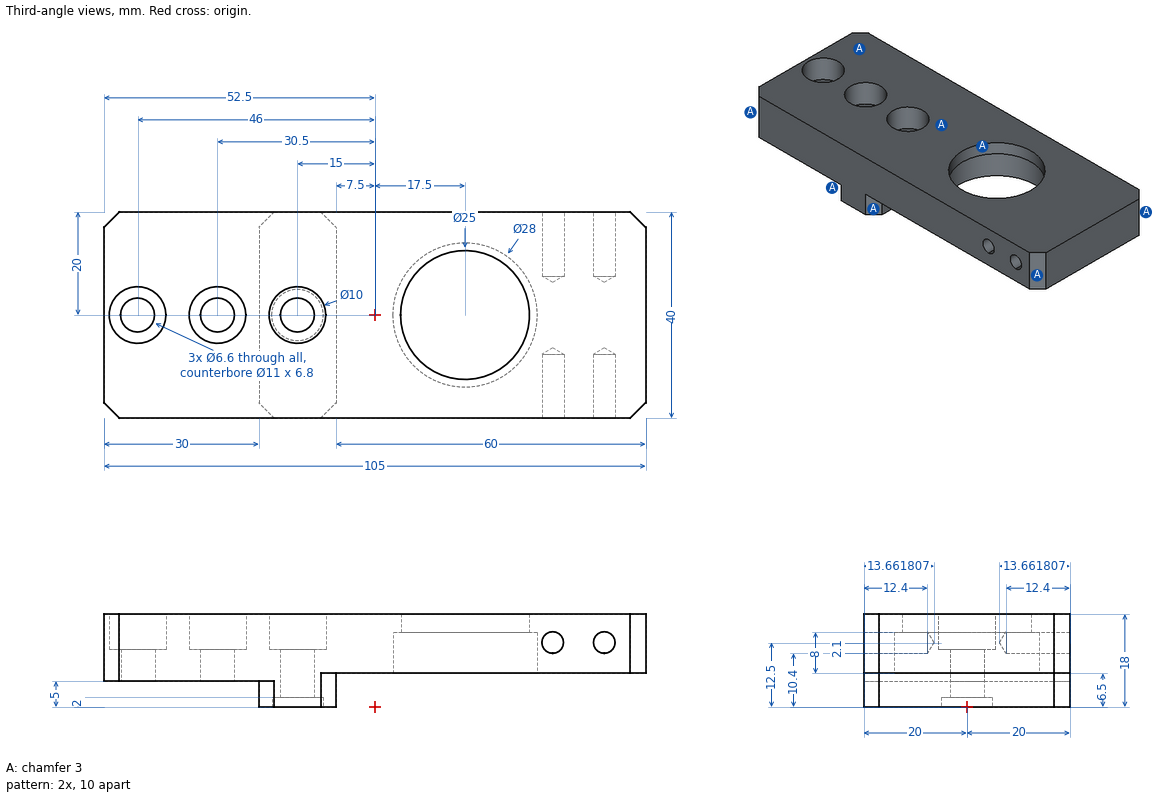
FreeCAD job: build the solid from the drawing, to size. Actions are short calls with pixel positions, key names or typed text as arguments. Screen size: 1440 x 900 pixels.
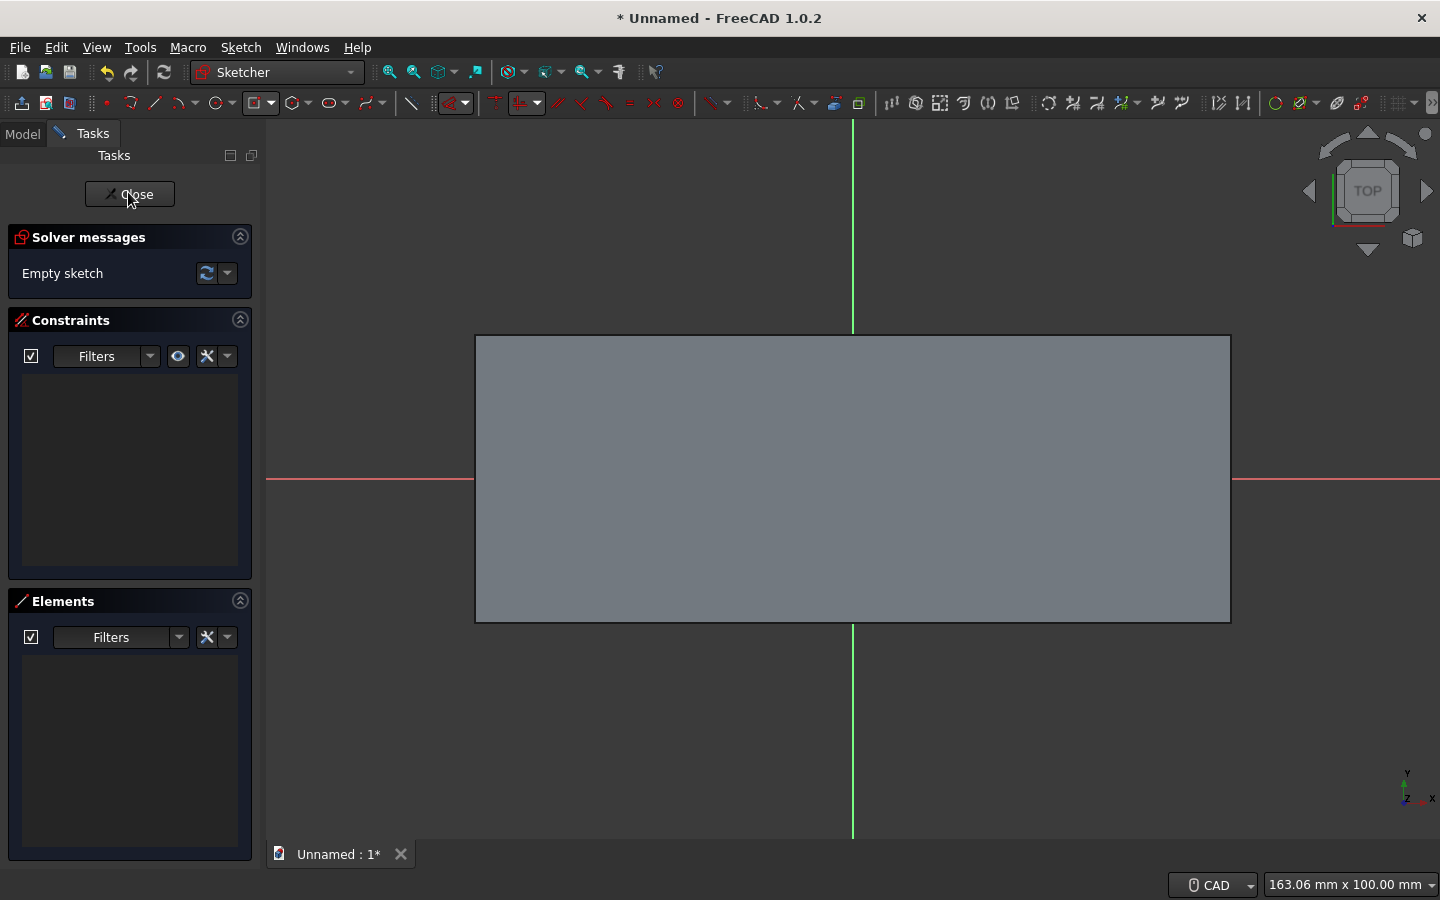
click(70, 104)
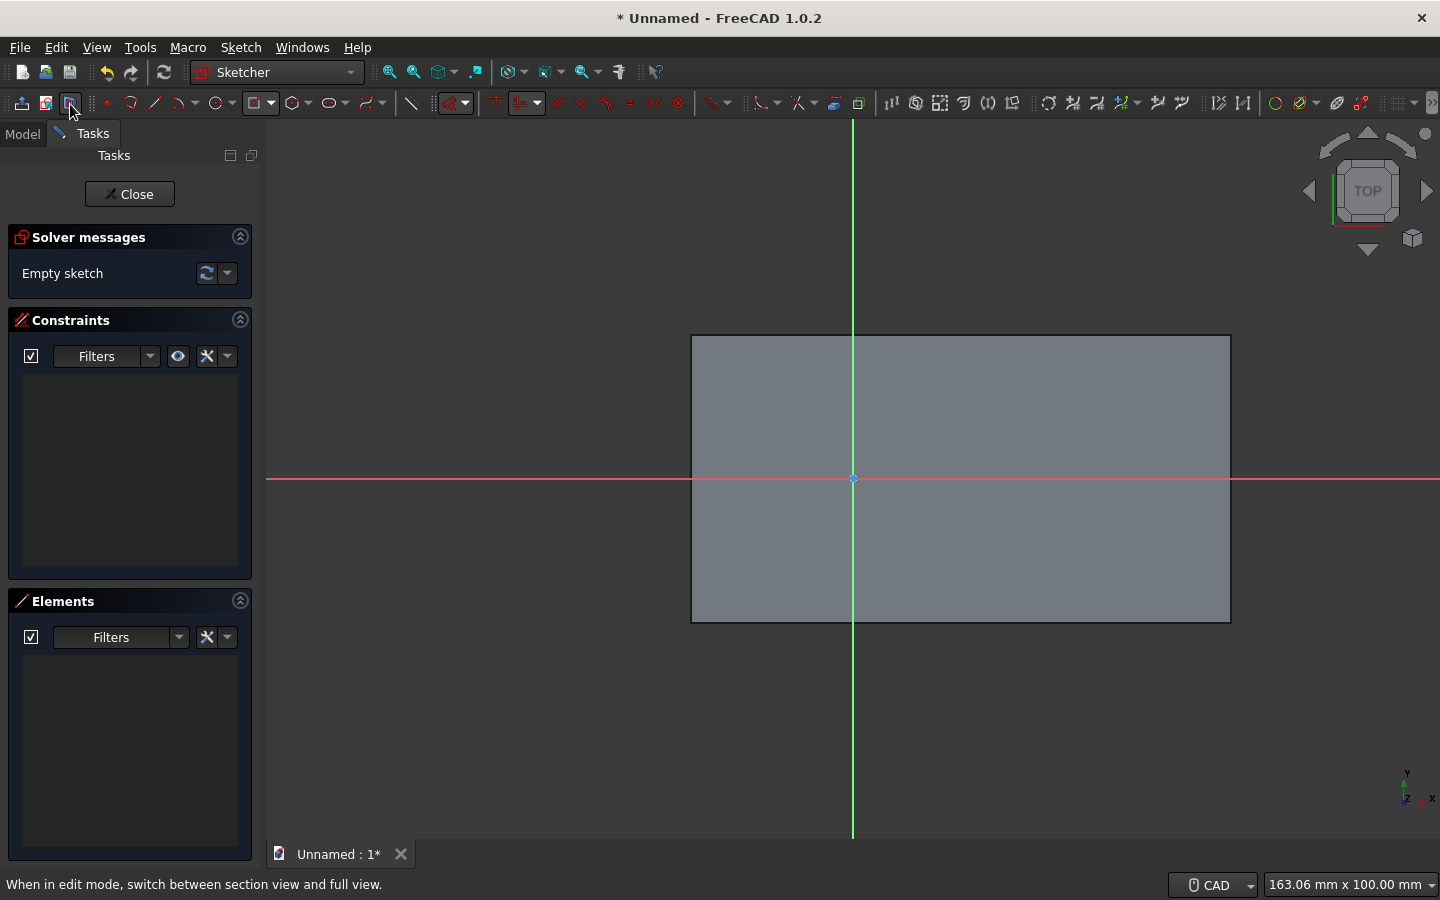
scroll(1275, 479, up, 2)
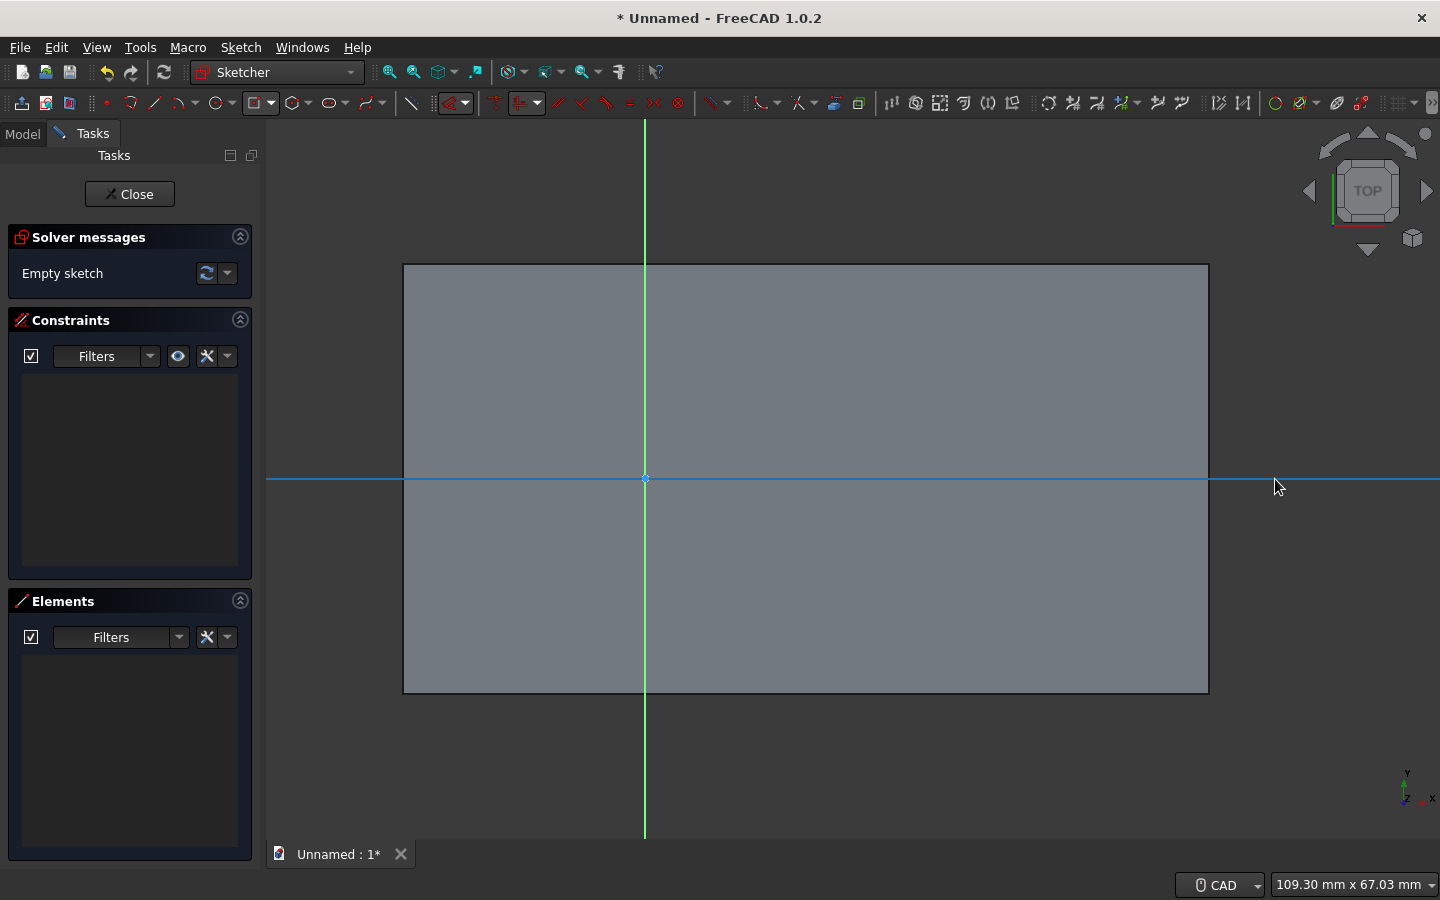
click(274, 104)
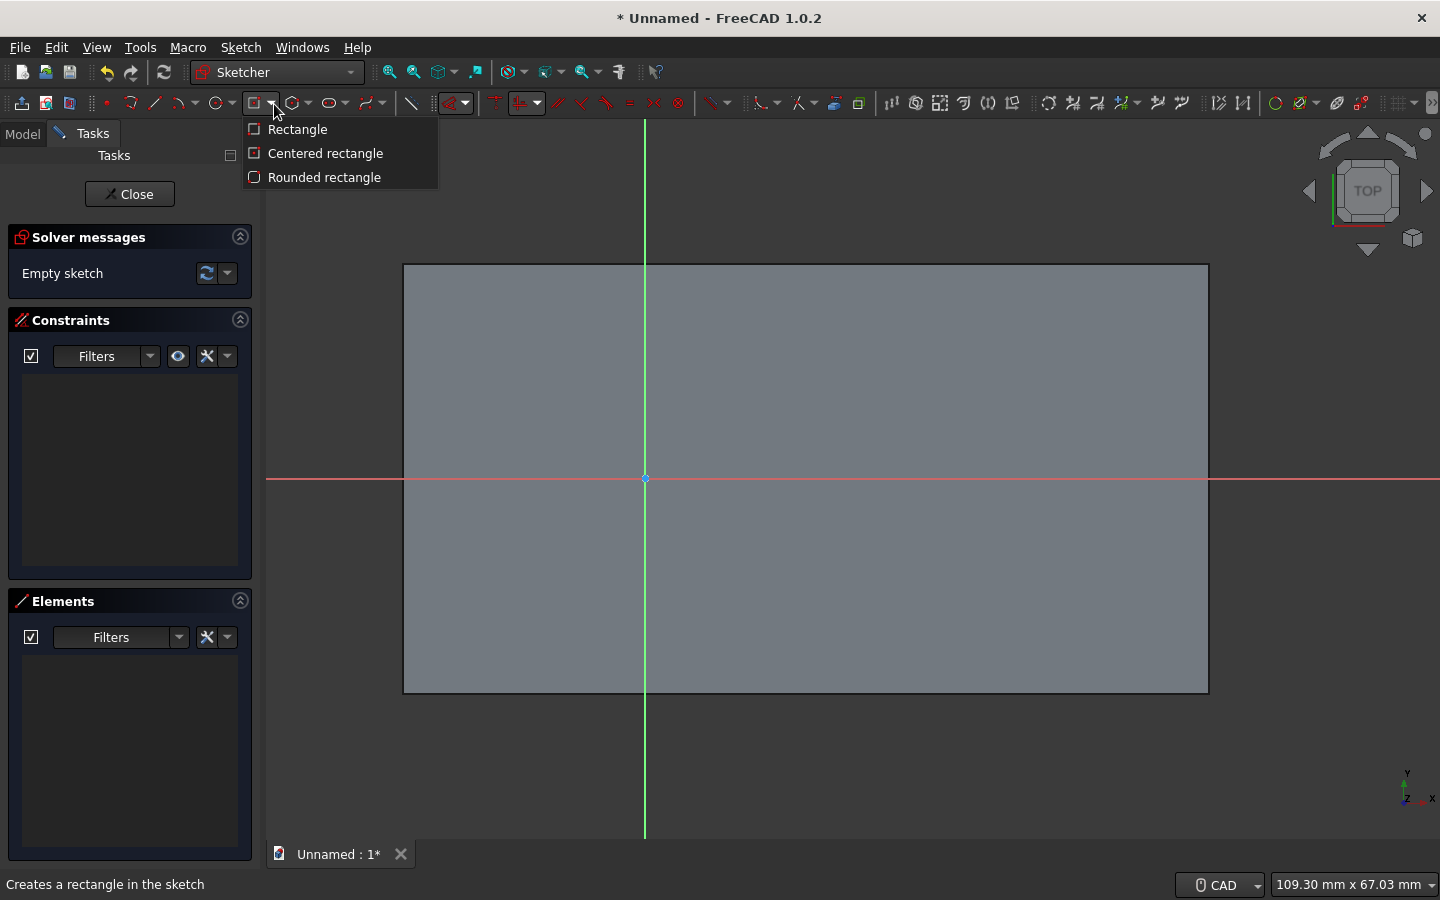
click(340, 129)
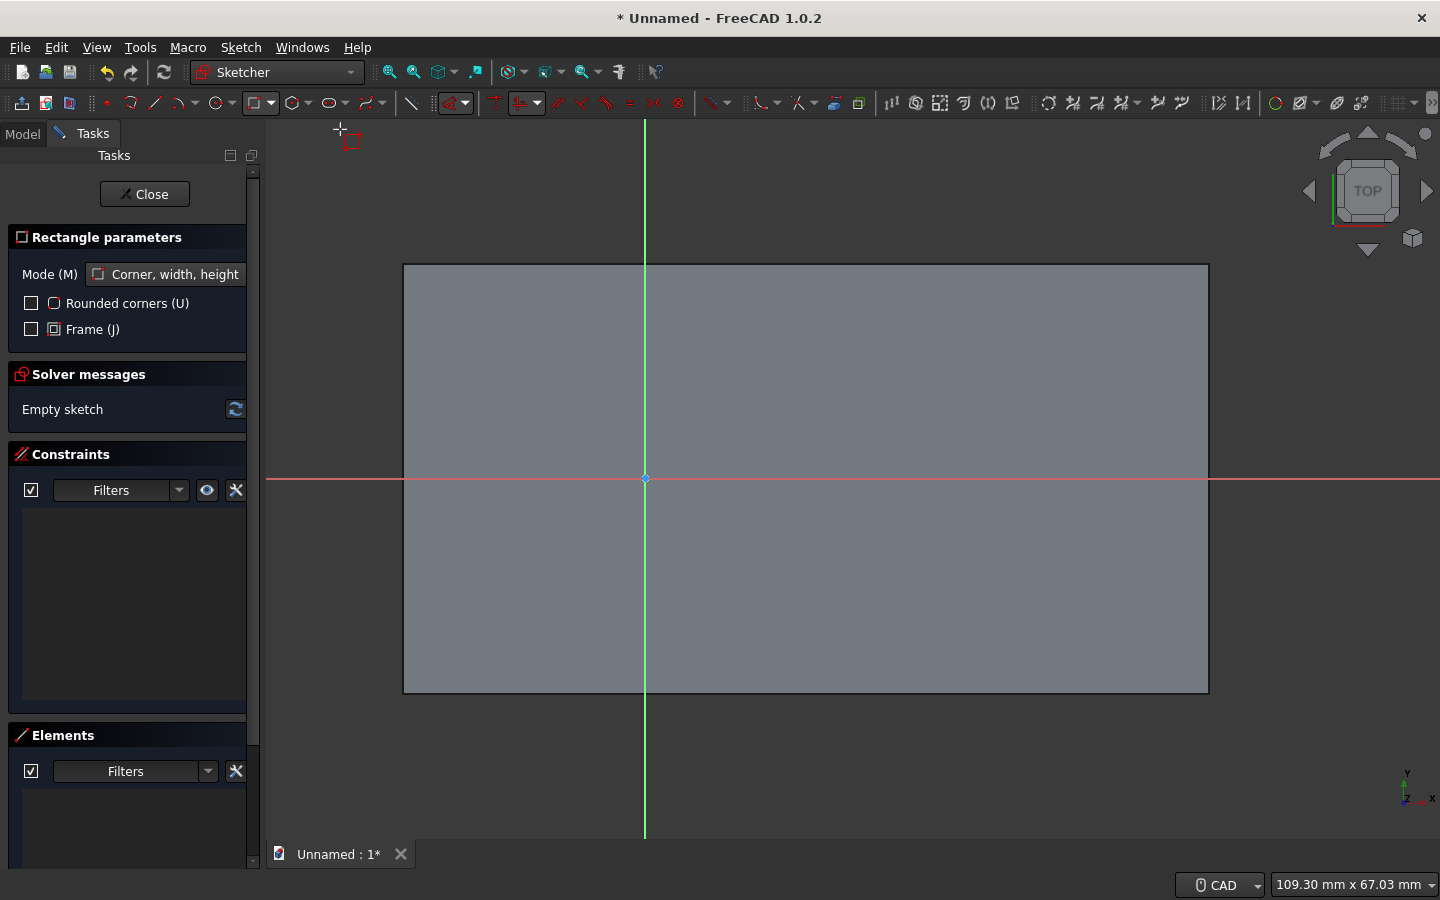
click(564, 264)
click(1209, 694)
key(Escape)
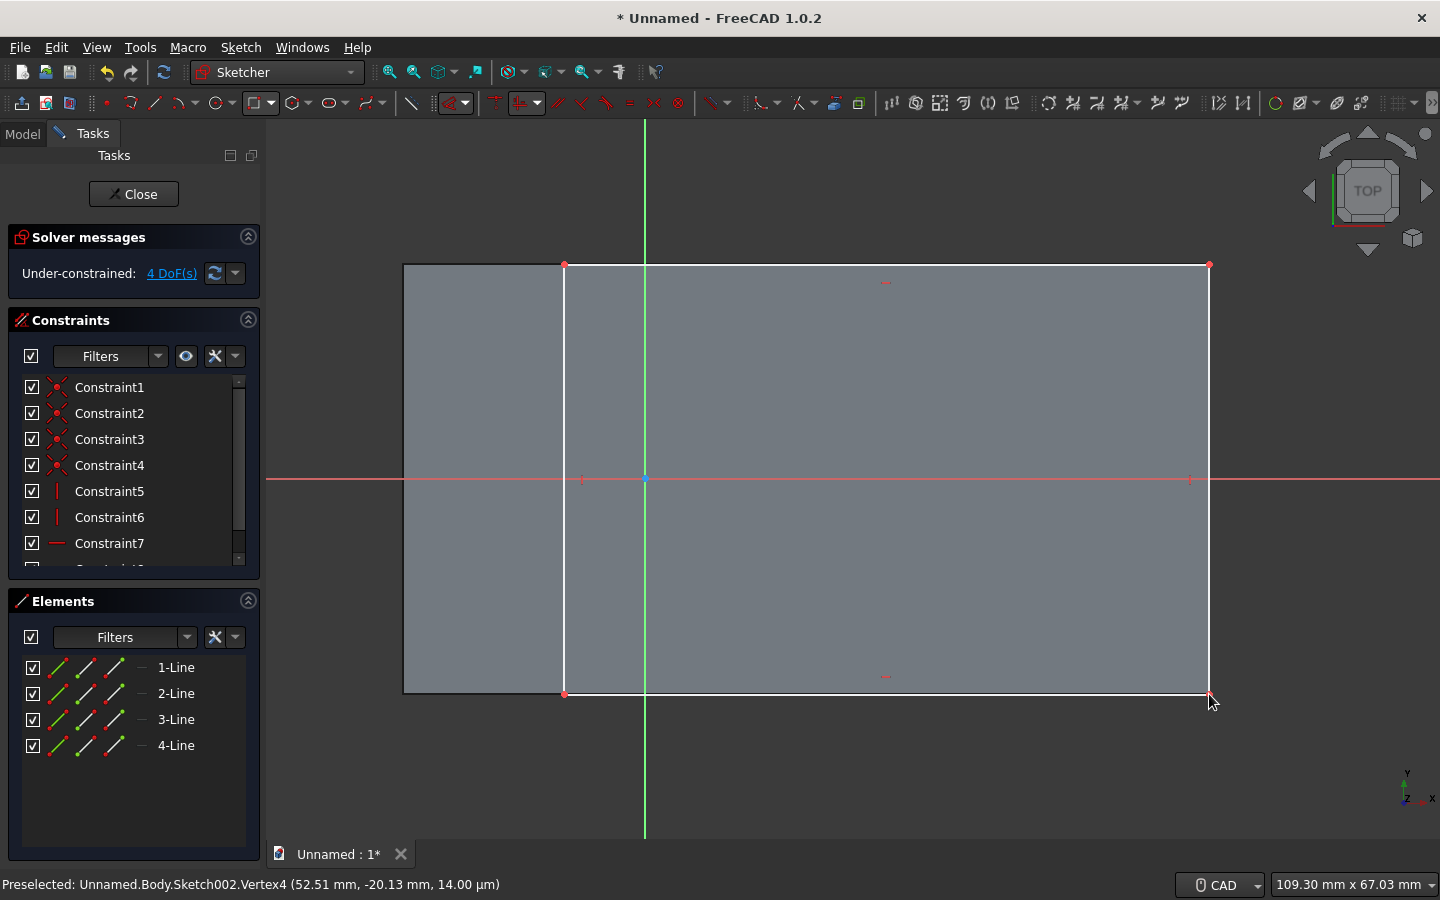
click(564, 394)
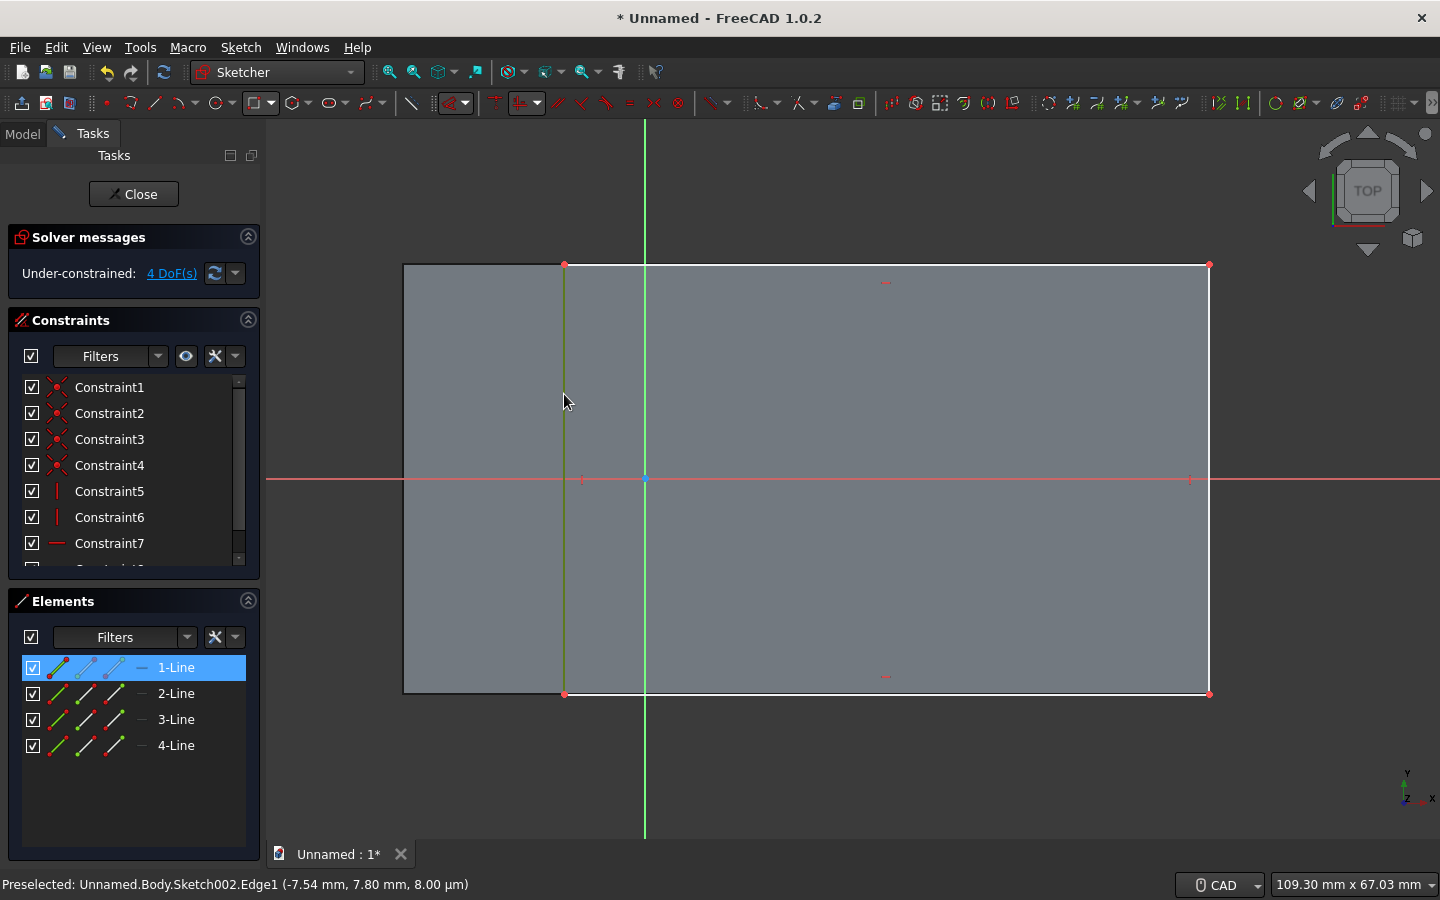
key(i)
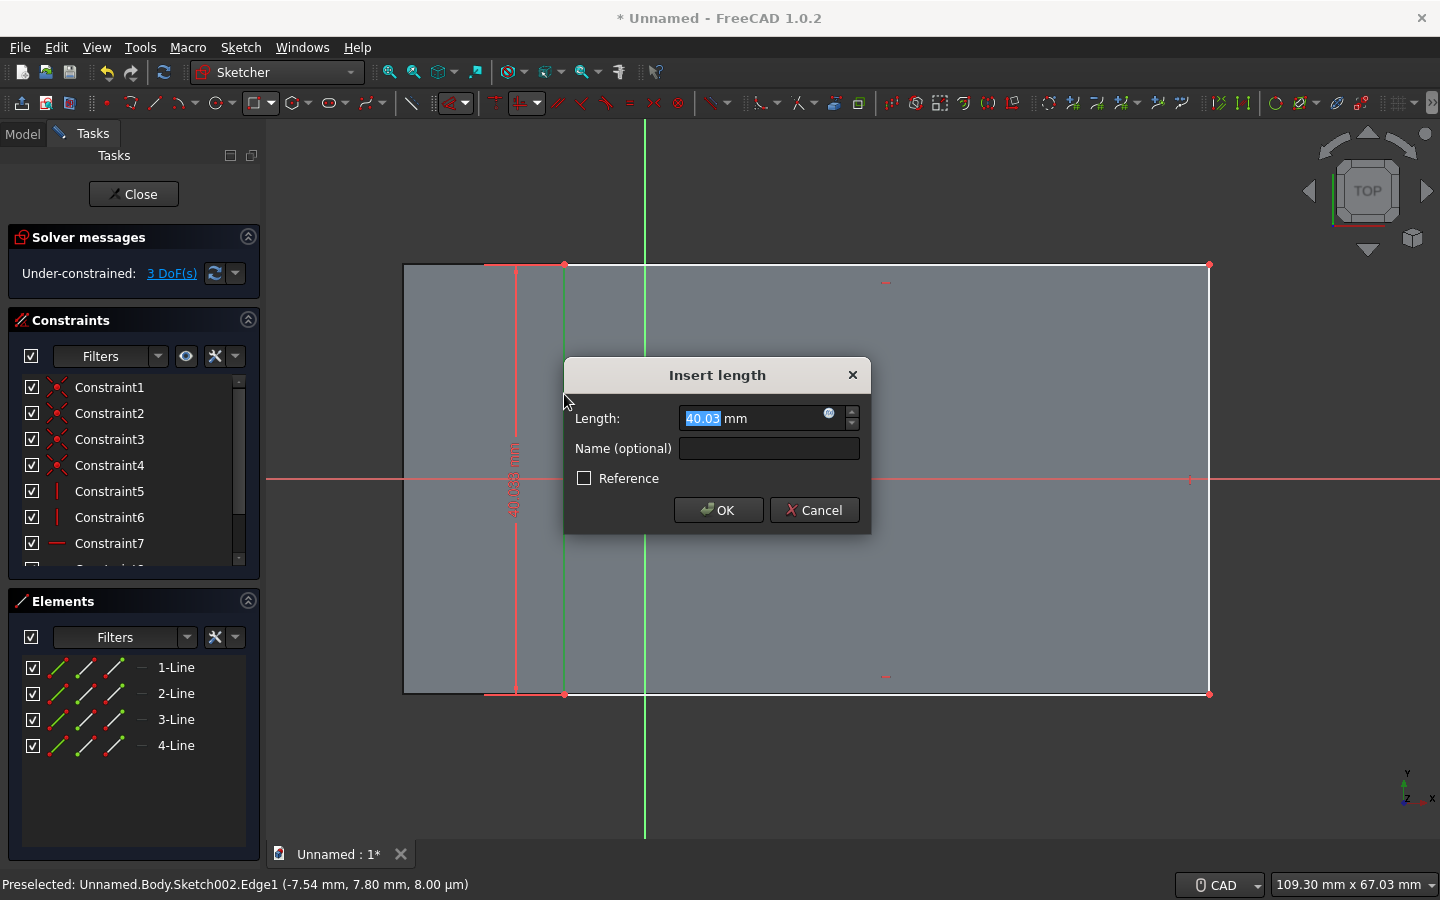
text(40)
key(Return)